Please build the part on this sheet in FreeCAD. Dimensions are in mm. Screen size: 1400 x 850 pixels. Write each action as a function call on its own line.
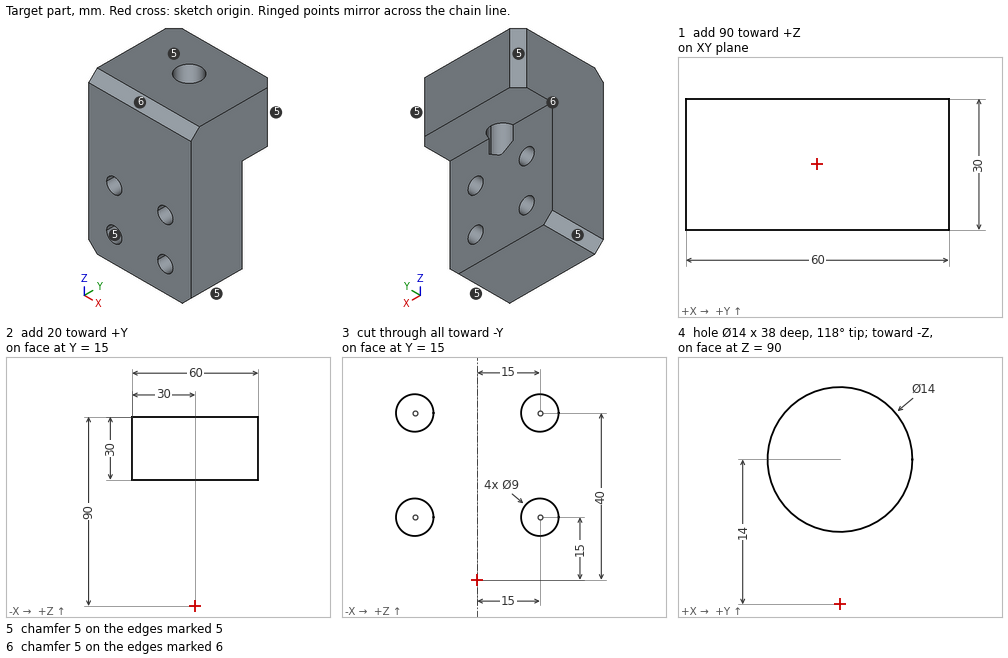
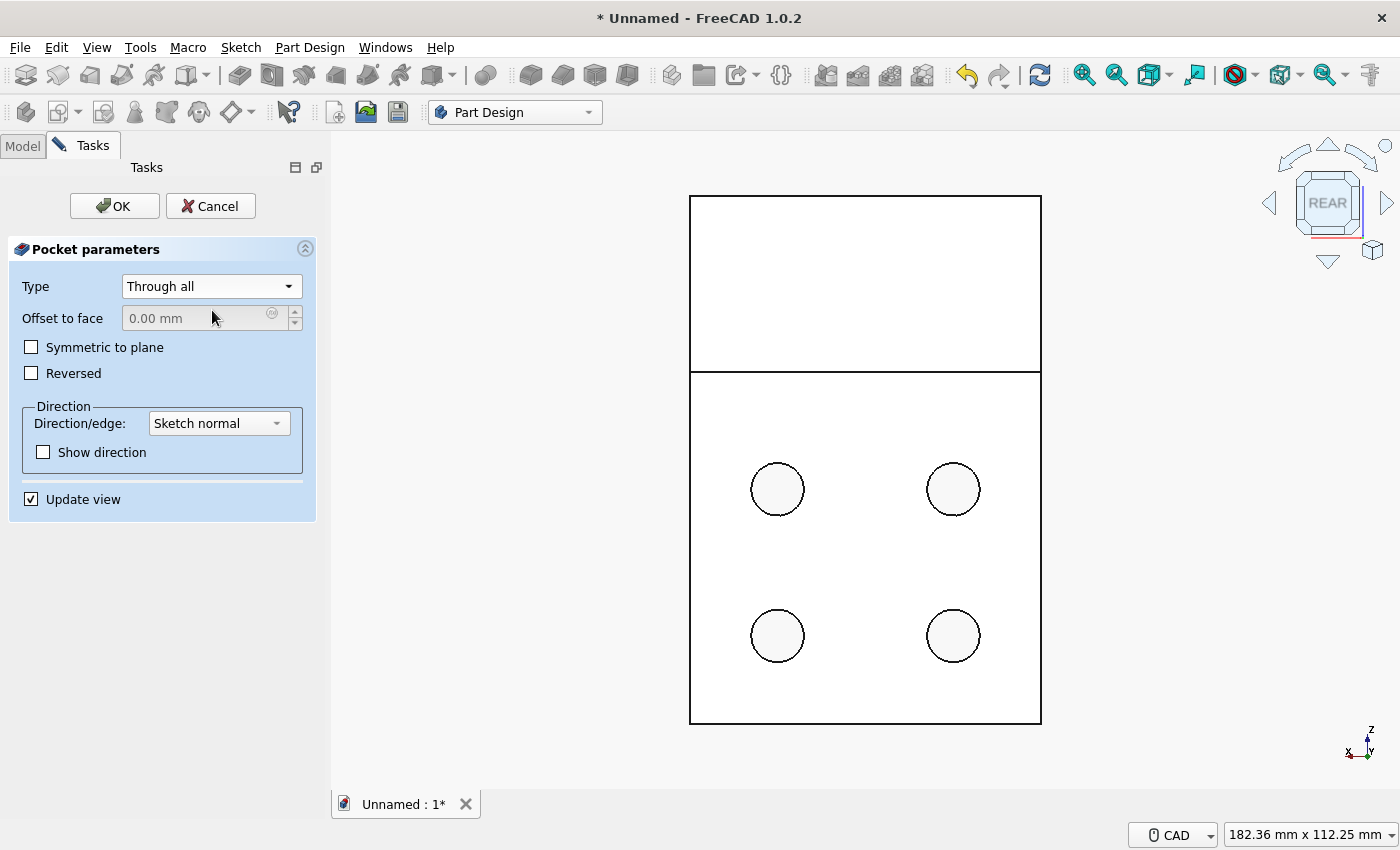
click(115, 206)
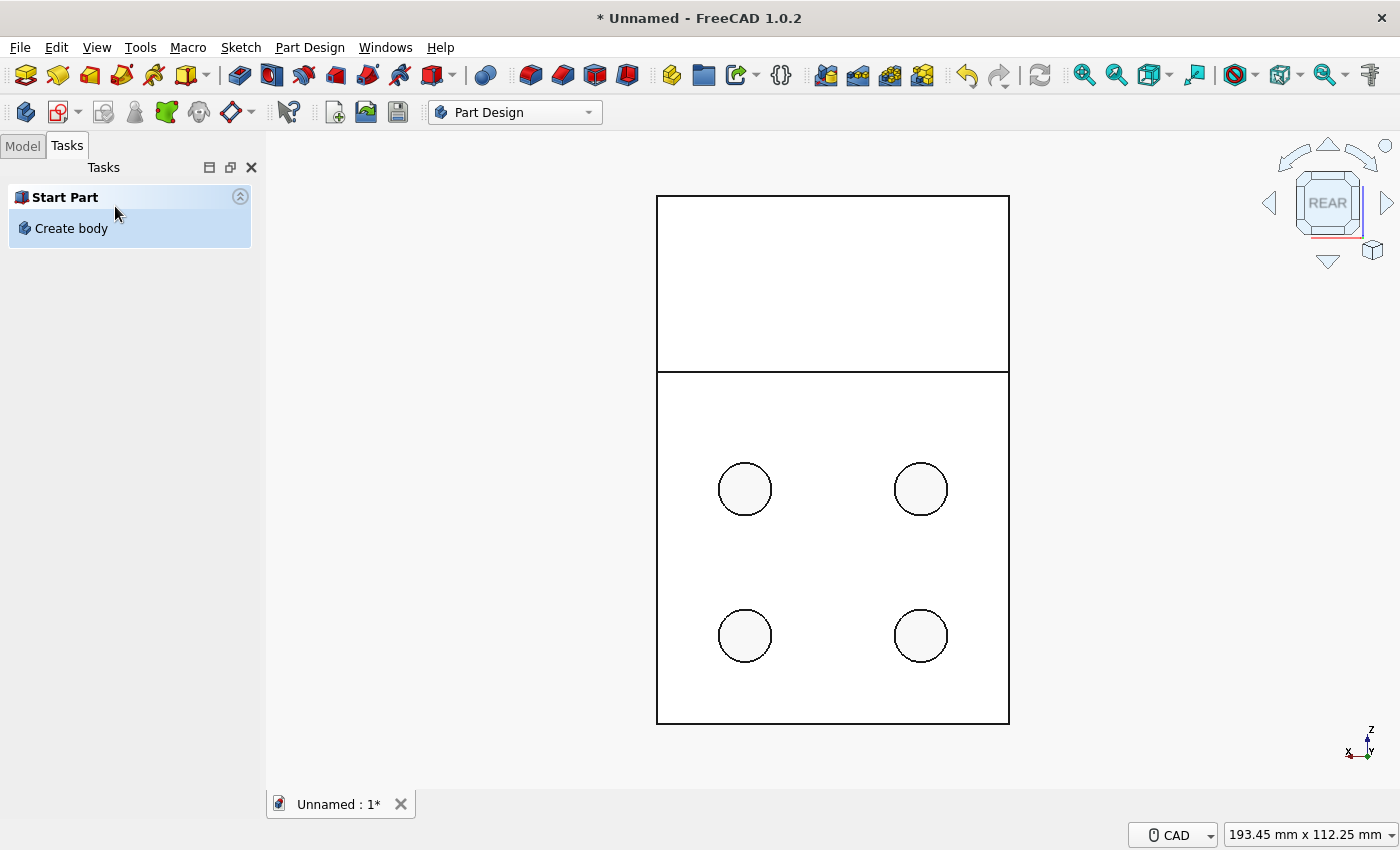
key(0)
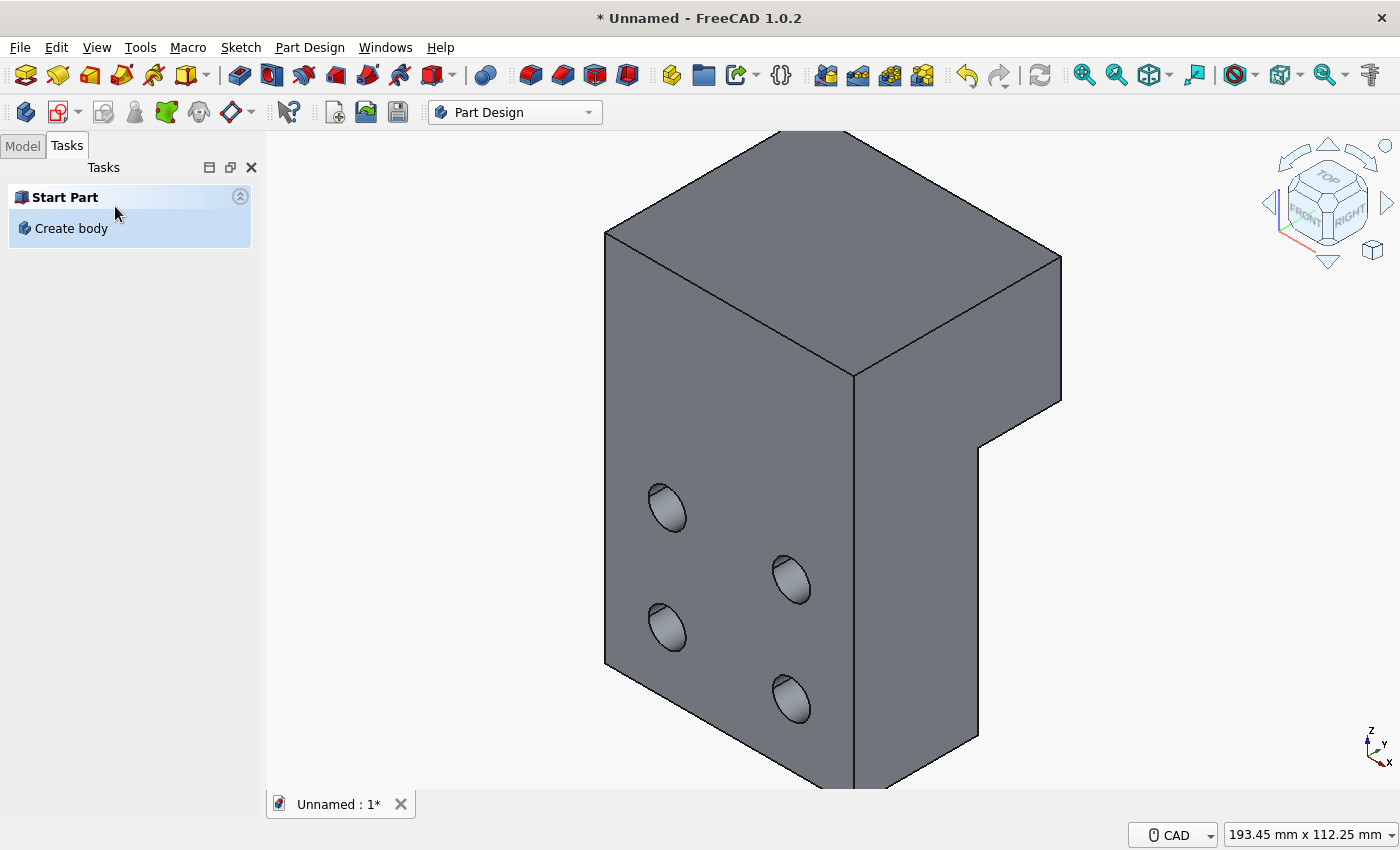
key(v)
key(f)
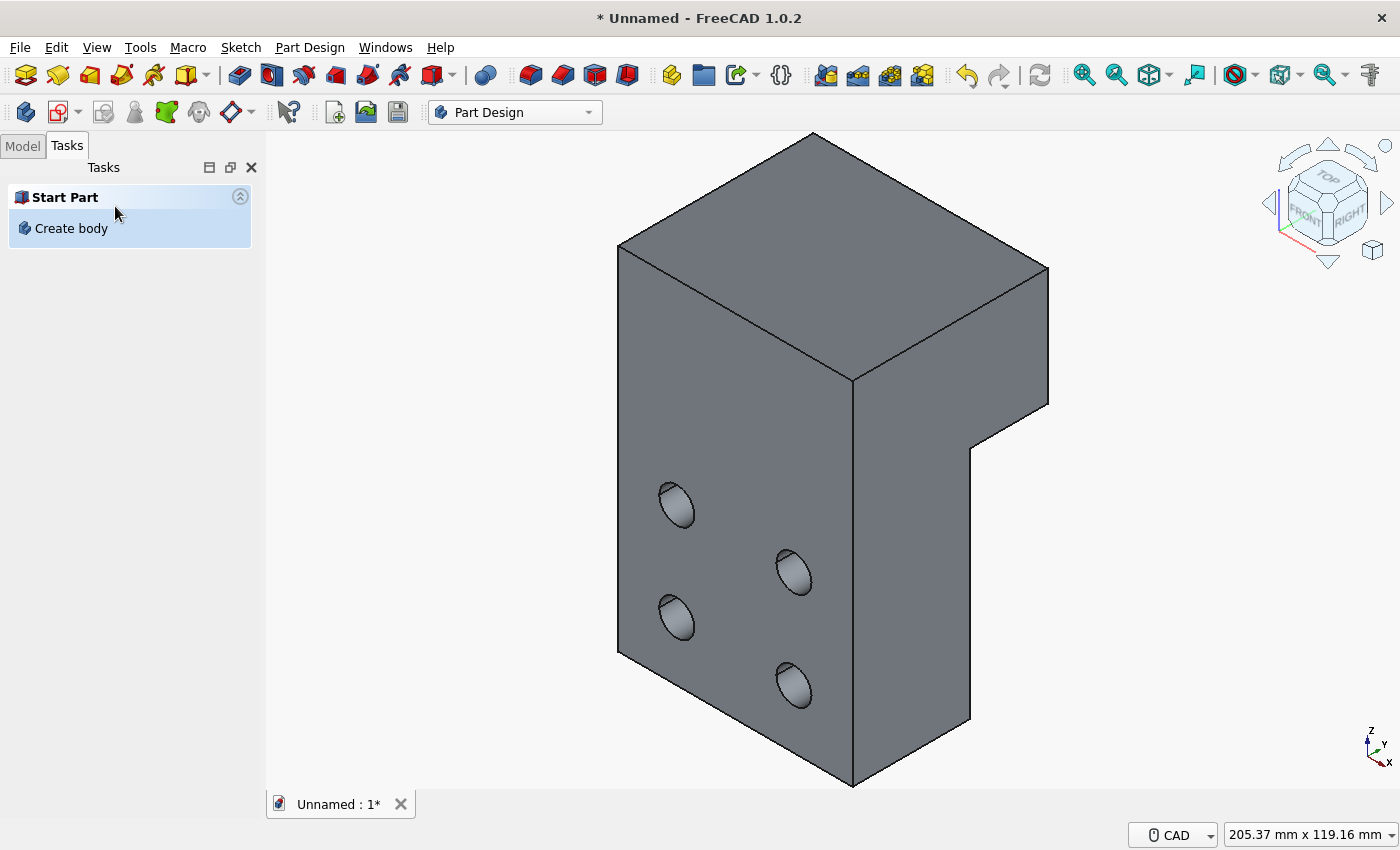
click(833, 256)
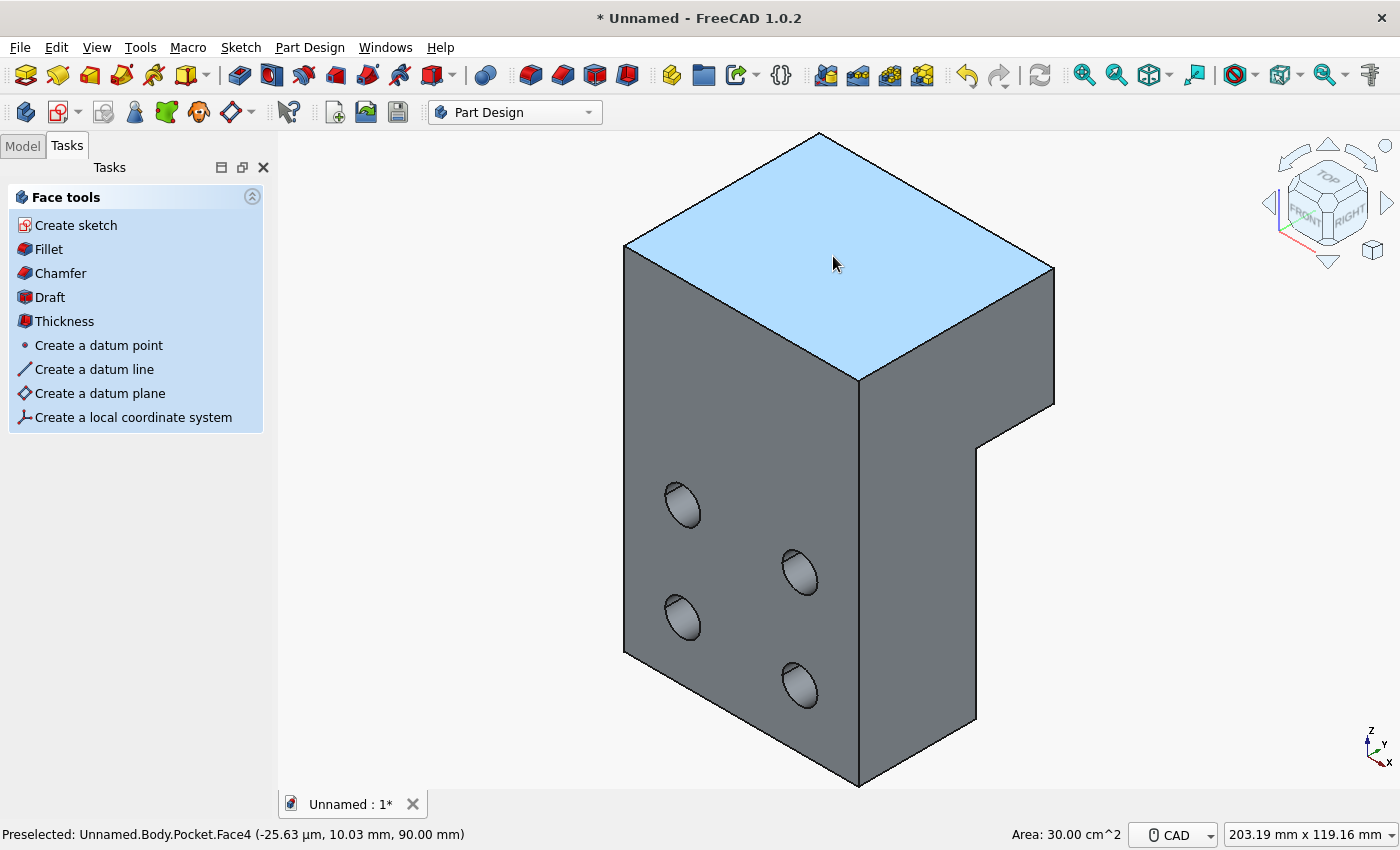
click(58, 112)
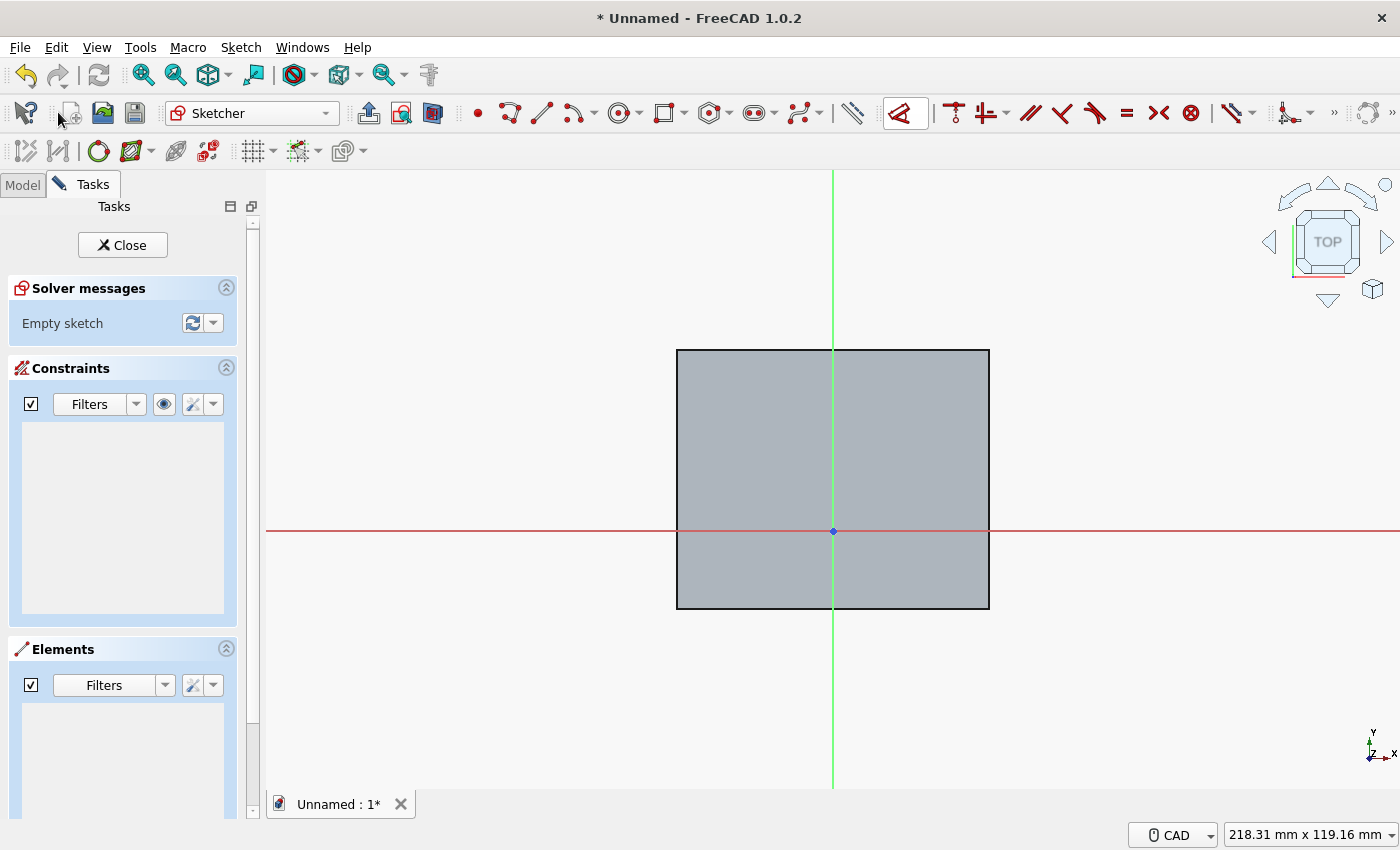
scroll(863, 476, up, 6)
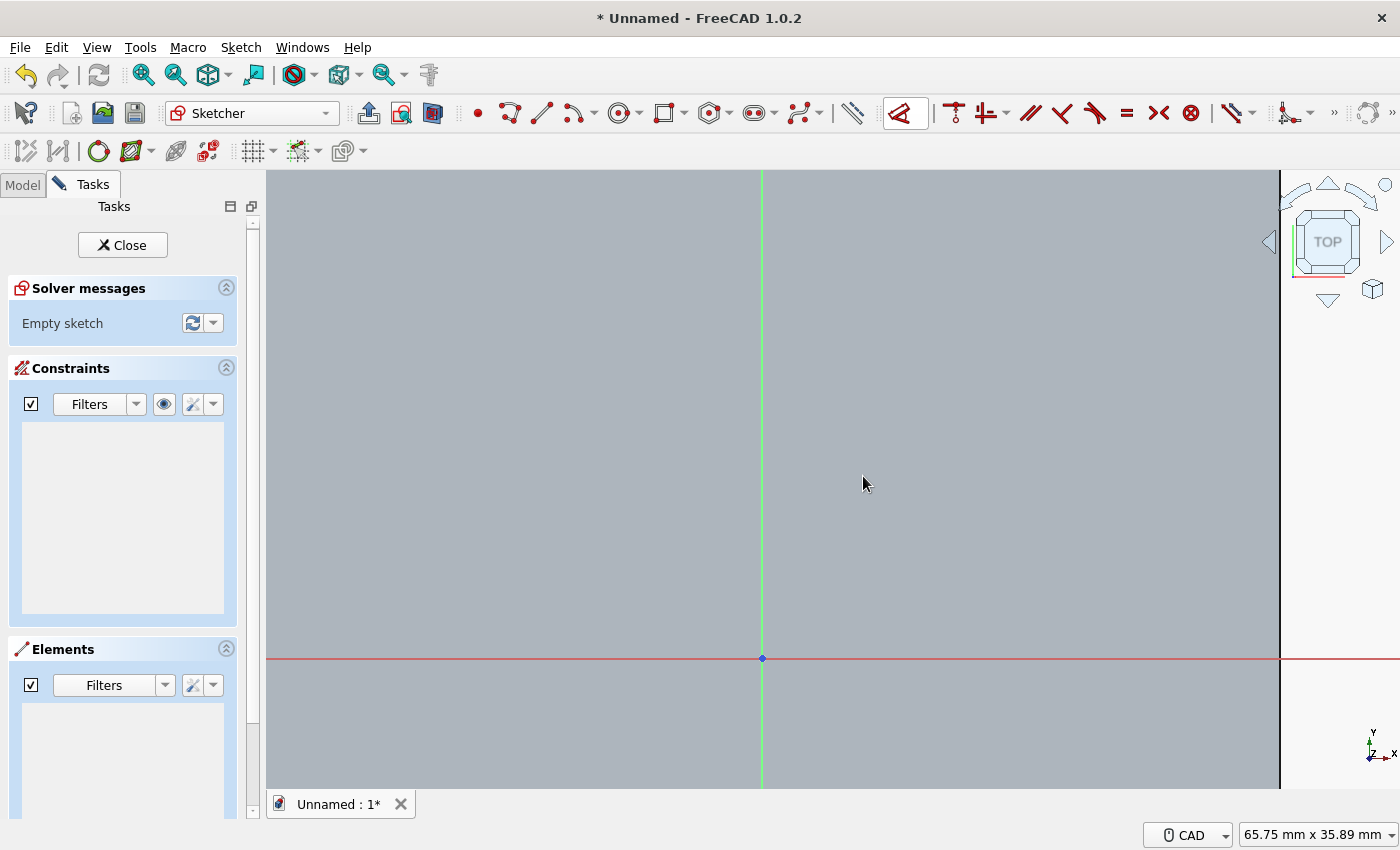
click(620, 114)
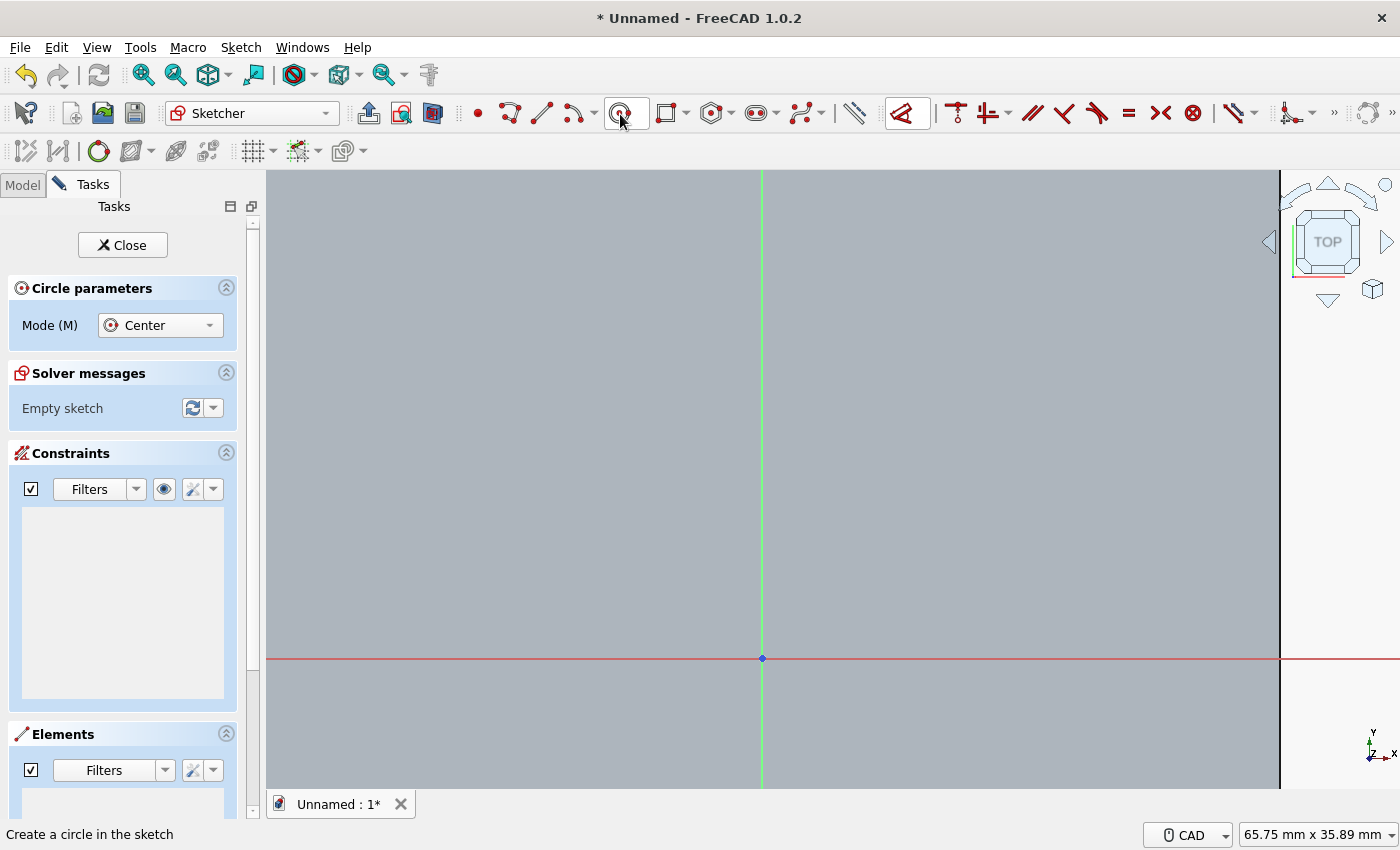
click(762, 417)
click(848, 332)
key(Escape)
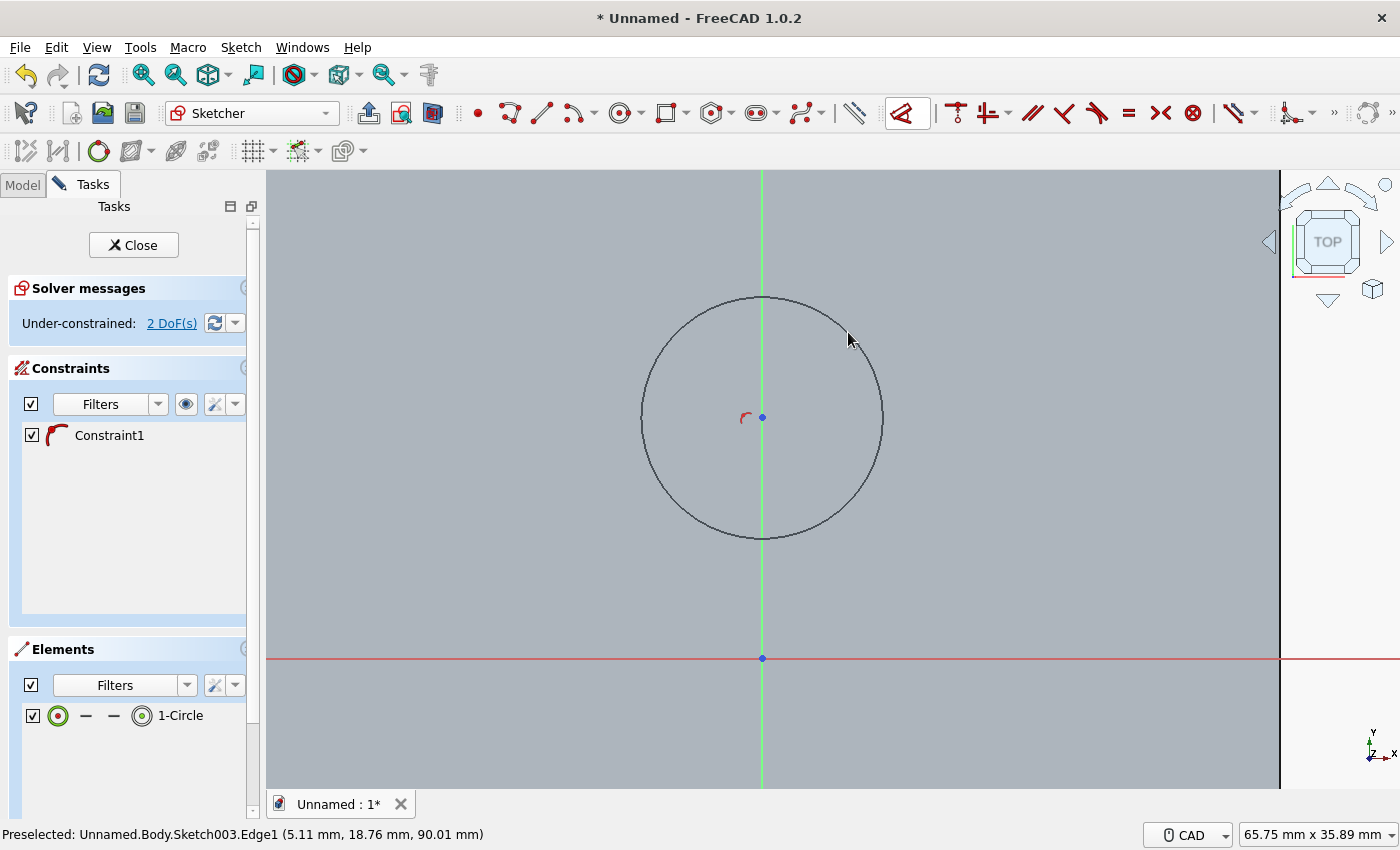
click(847, 332)